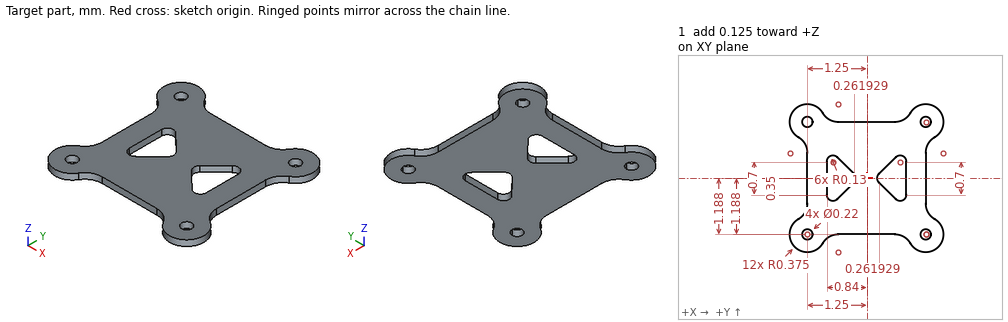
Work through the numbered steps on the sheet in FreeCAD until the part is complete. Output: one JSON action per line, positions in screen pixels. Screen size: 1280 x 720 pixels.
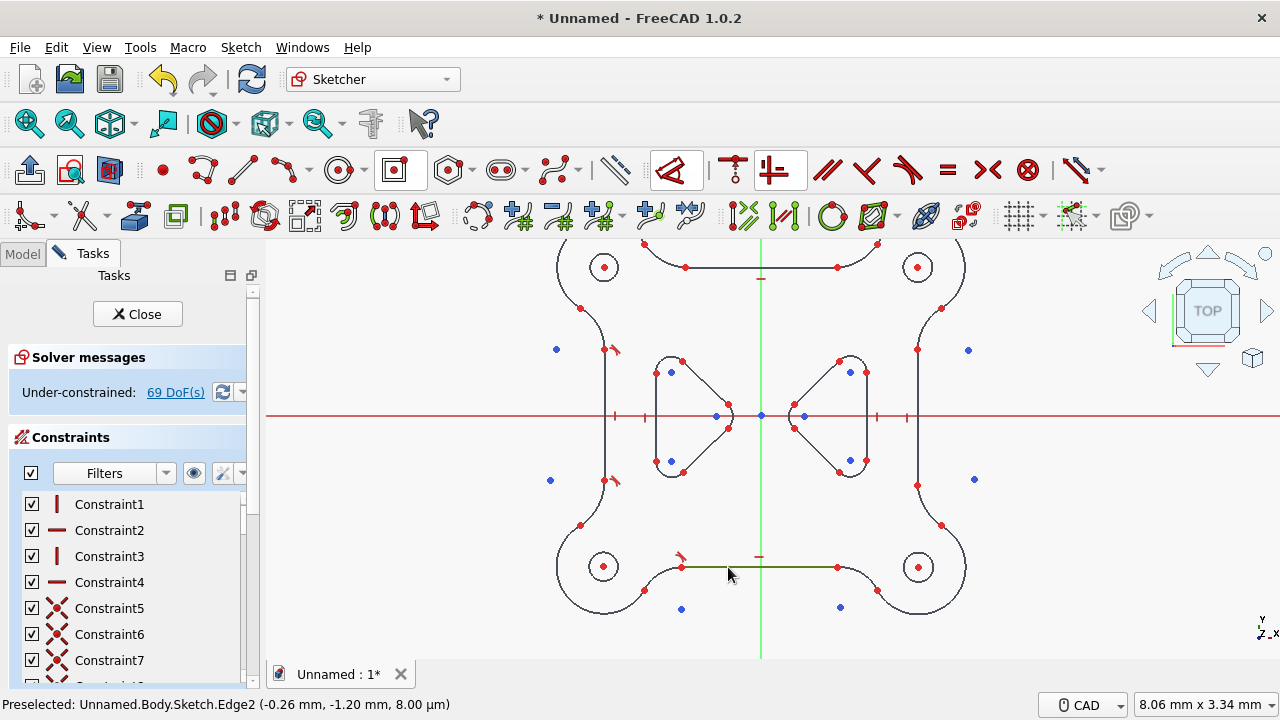
{"action": "left_click", "coordinate": [869, 578]}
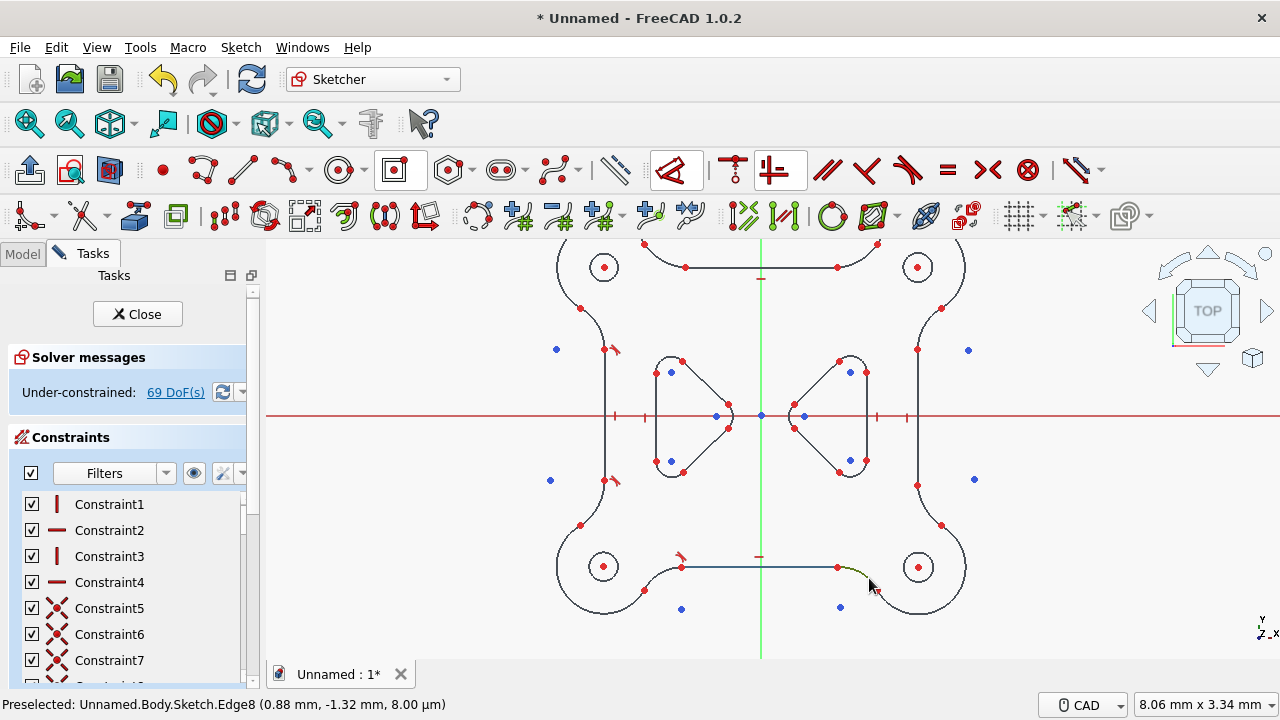
{"action": "left_click", "coordinate": [908, 170]}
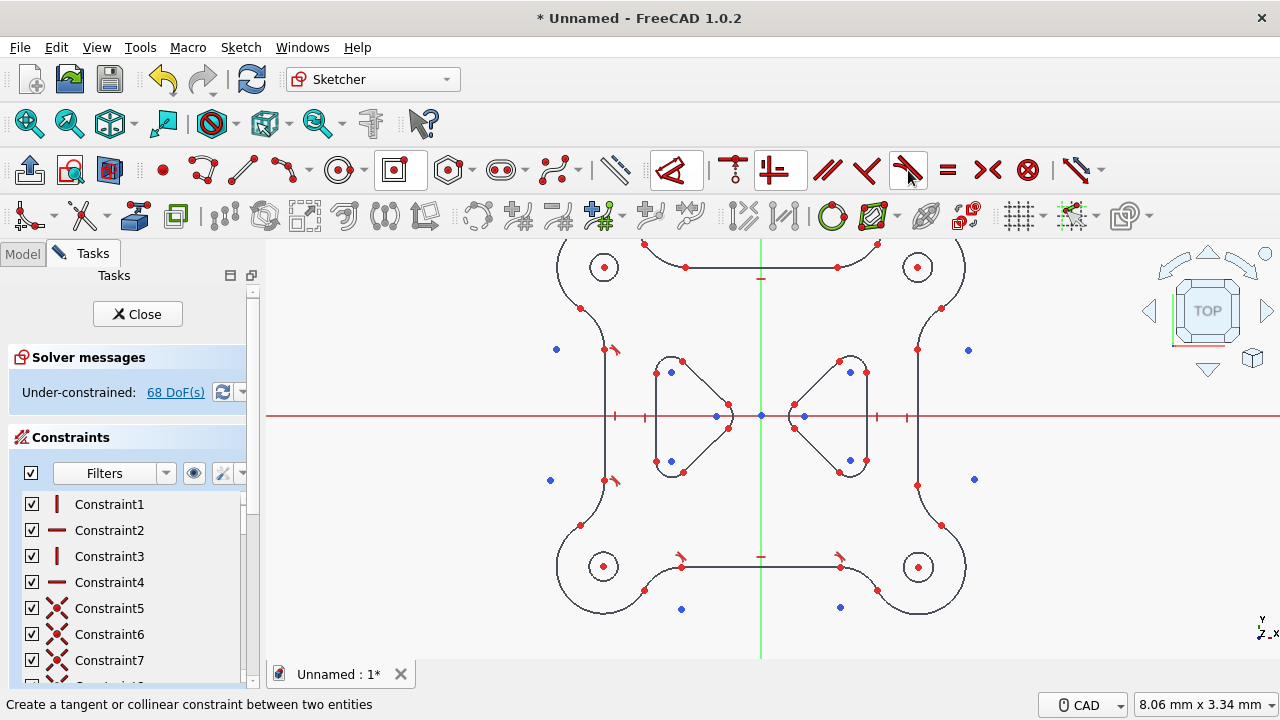
{"action": "left_click", "coordinate": [918, 445]}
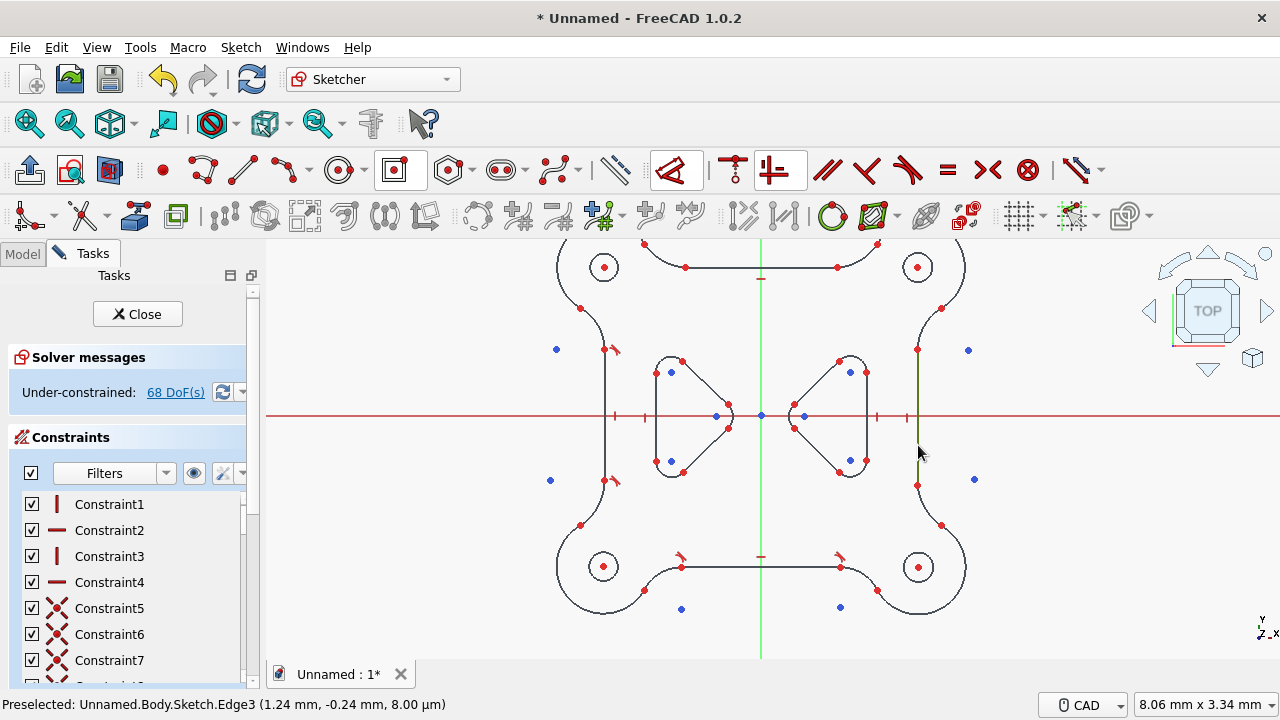
{"action": "left_click", "coordinate": [921, 500]}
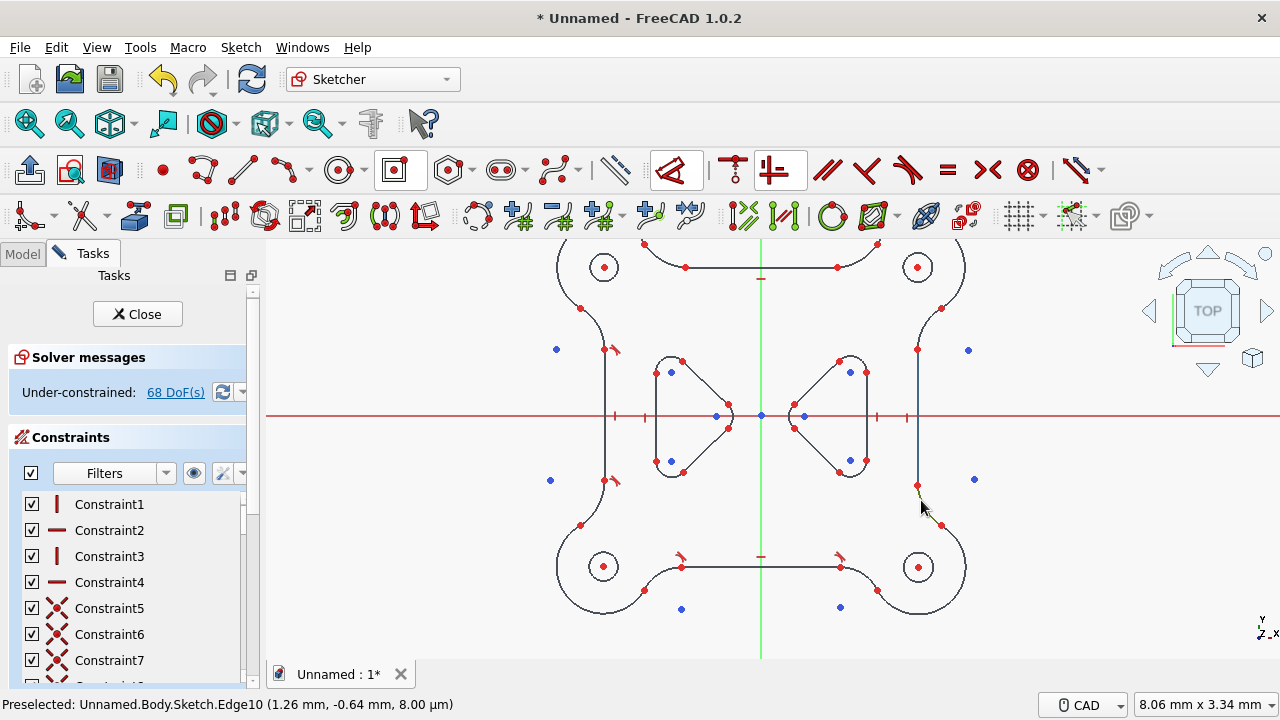
{"action": "left_click", "coordinate": [908, 170]}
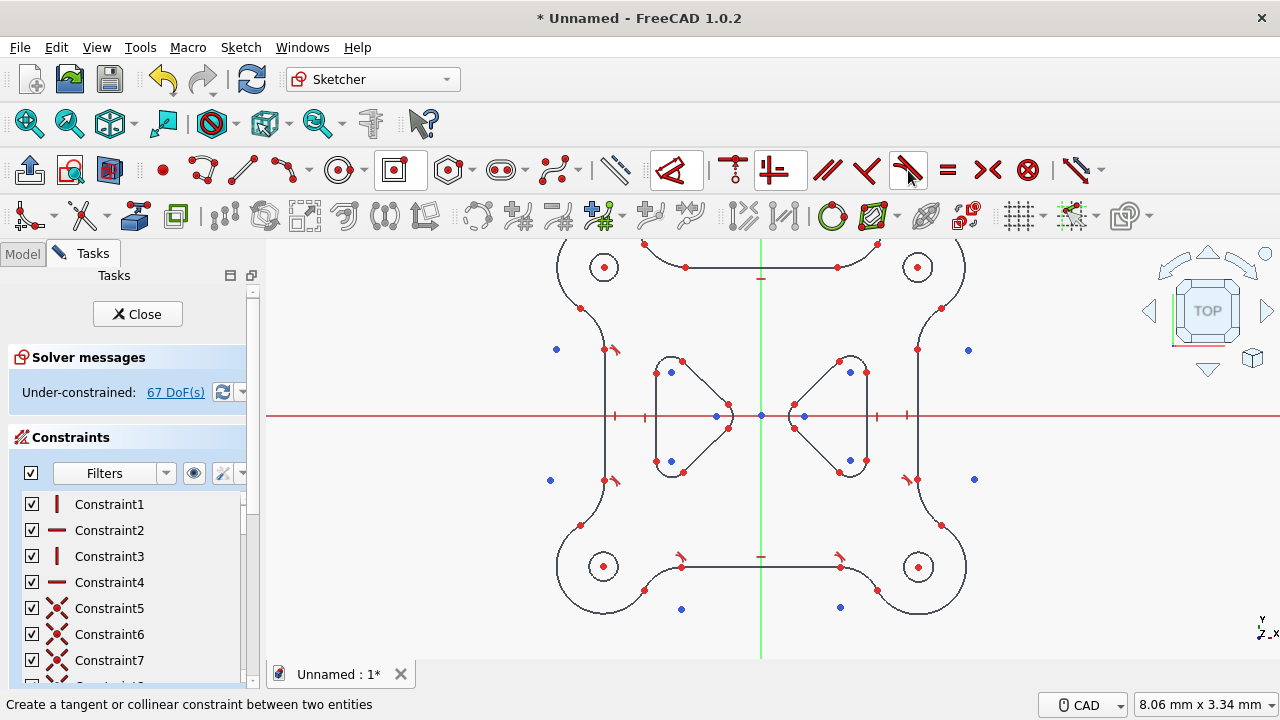
{"action": "left_click", "coordinate": [918, 440]}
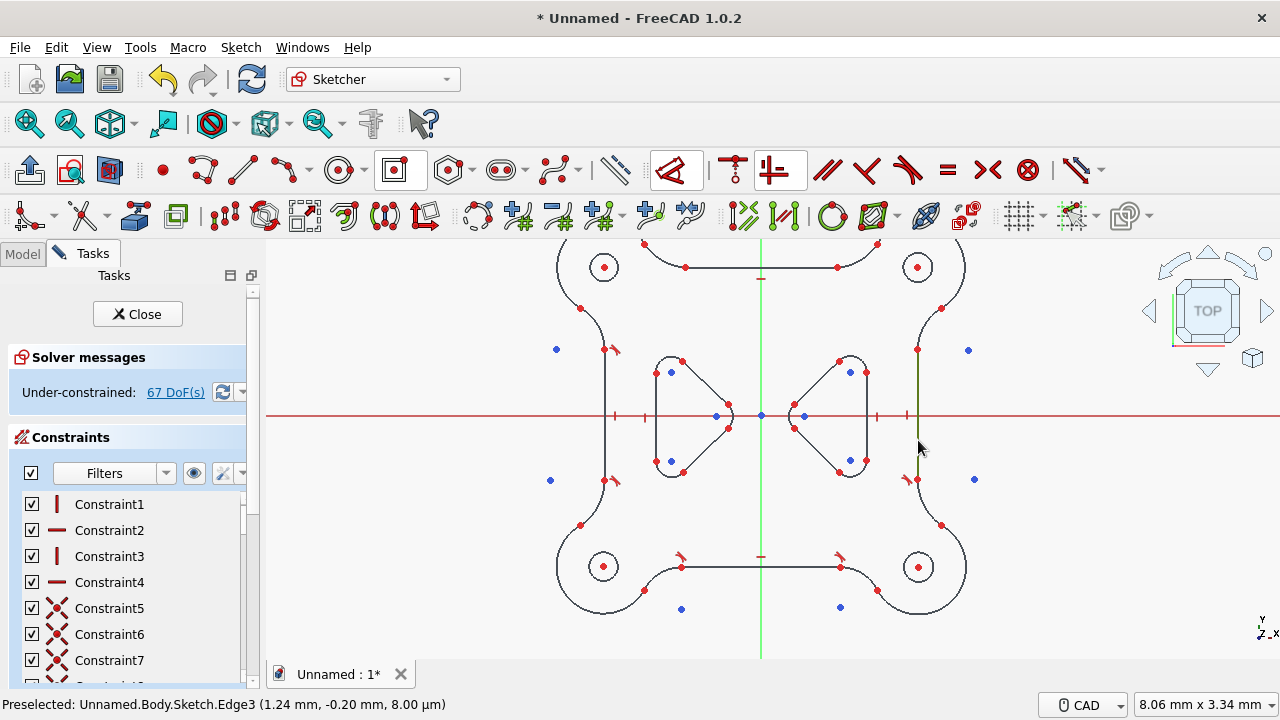
{"action": "left_click", "coordinate": [930, 318]}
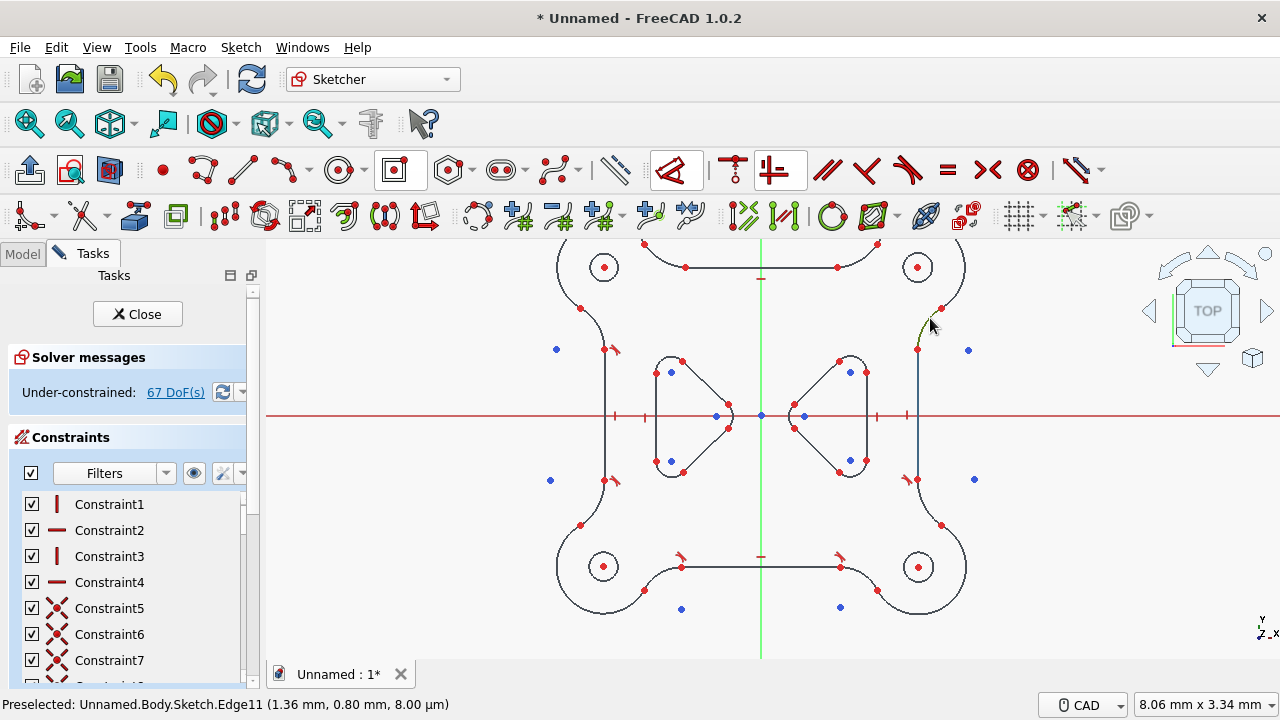
{"action": "left_click", "coordinate": [908, 170]}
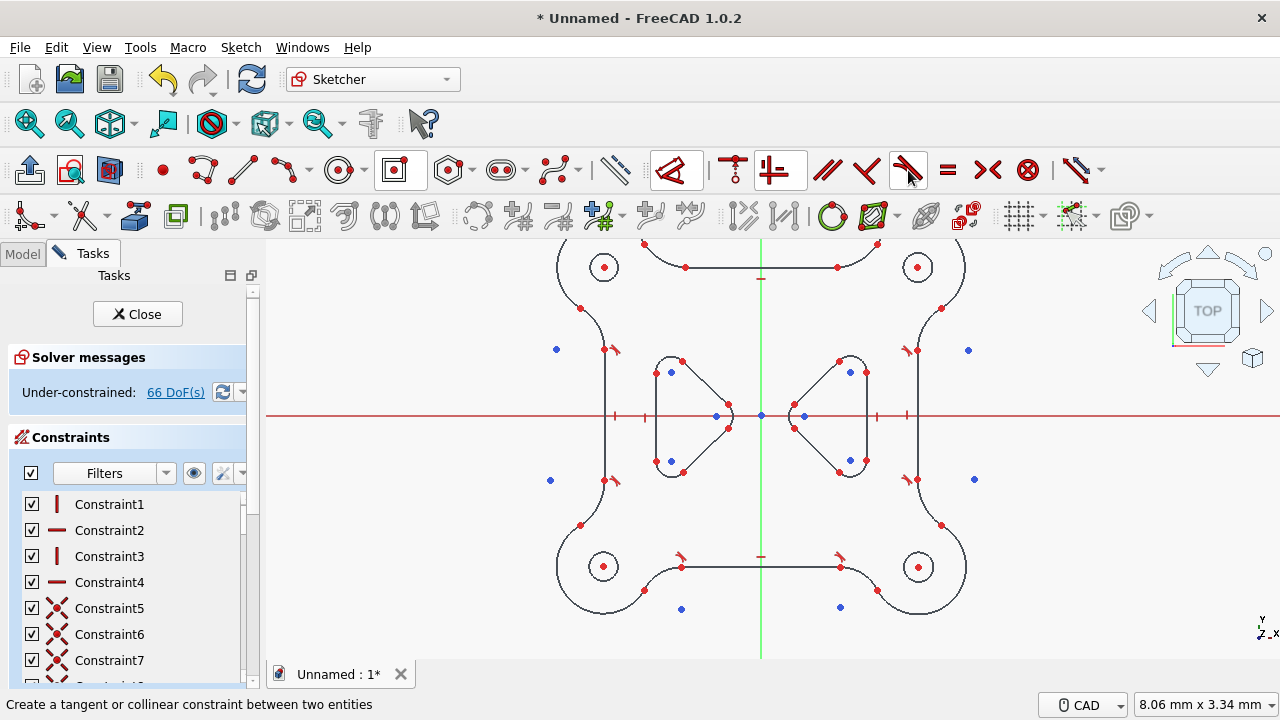
{"action": "left_click", "coordinate": [792, 268]}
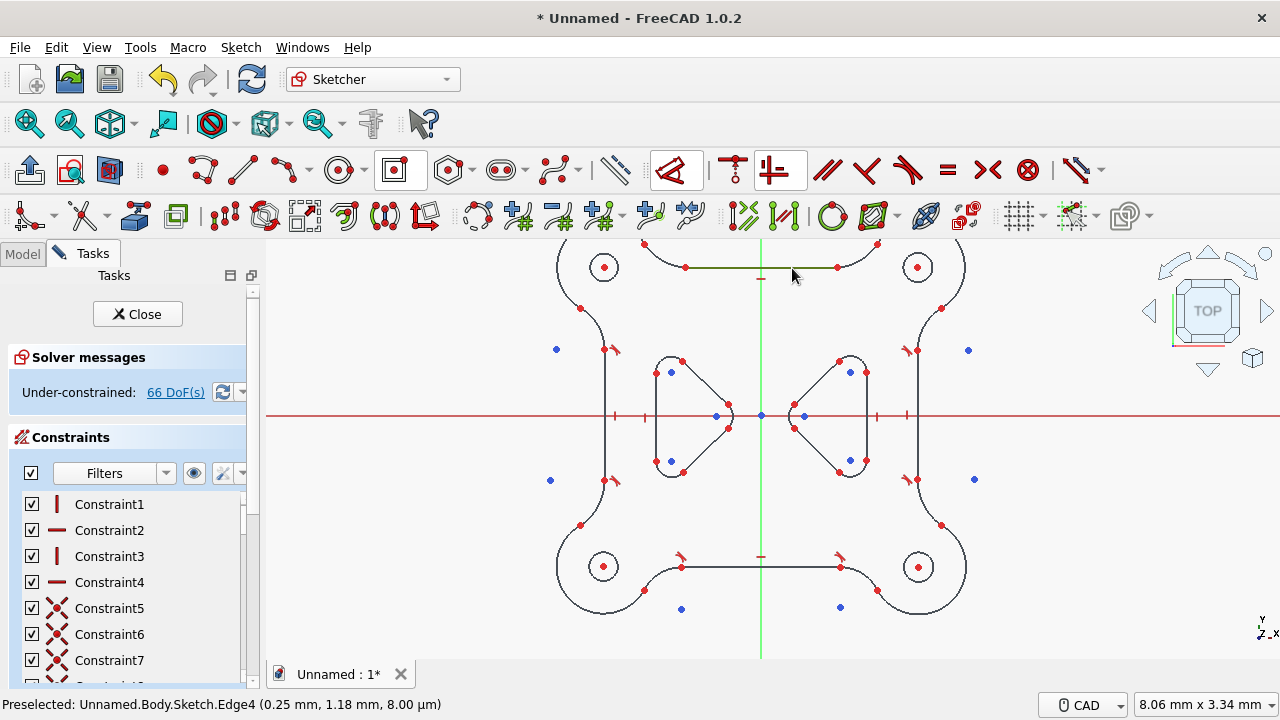
{"action": "scroll", "coordinate": [590, 516], "scroll_direction": "down", "scroll_amount": 2}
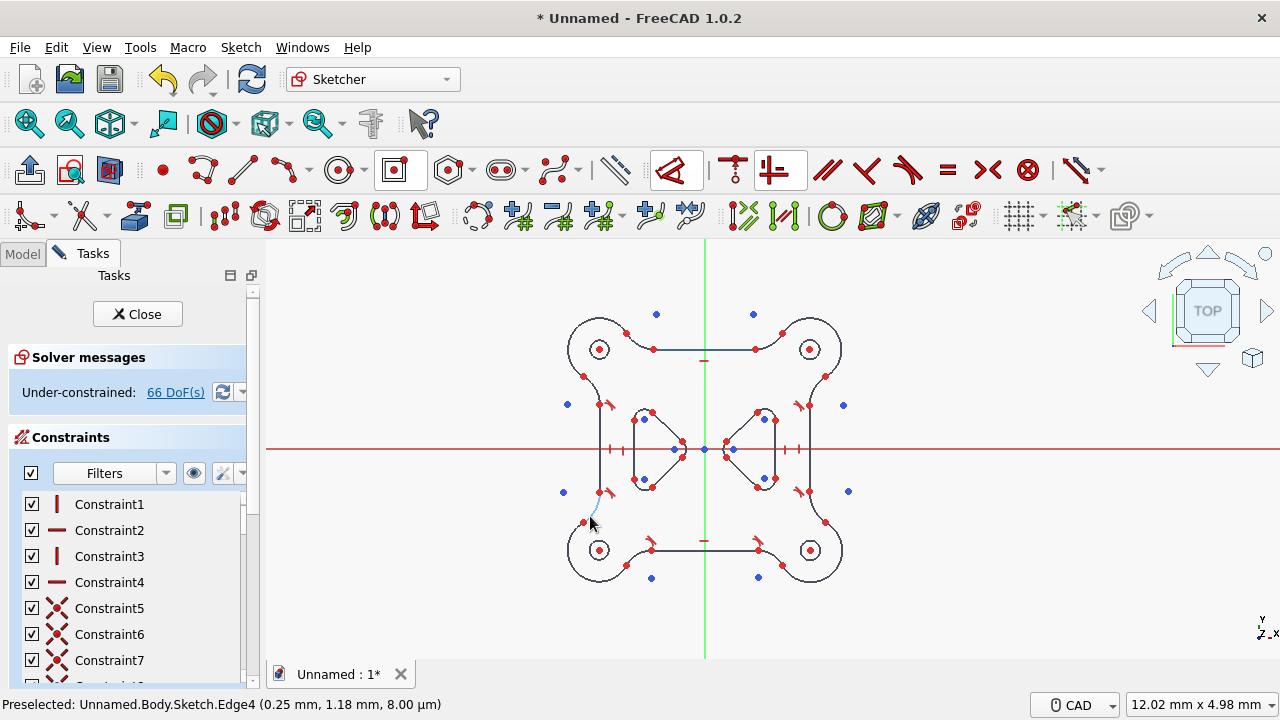
{"action": "scroll", "coordinate": [765, 348], "scroll_direction": "up", "scroll_amount": 2}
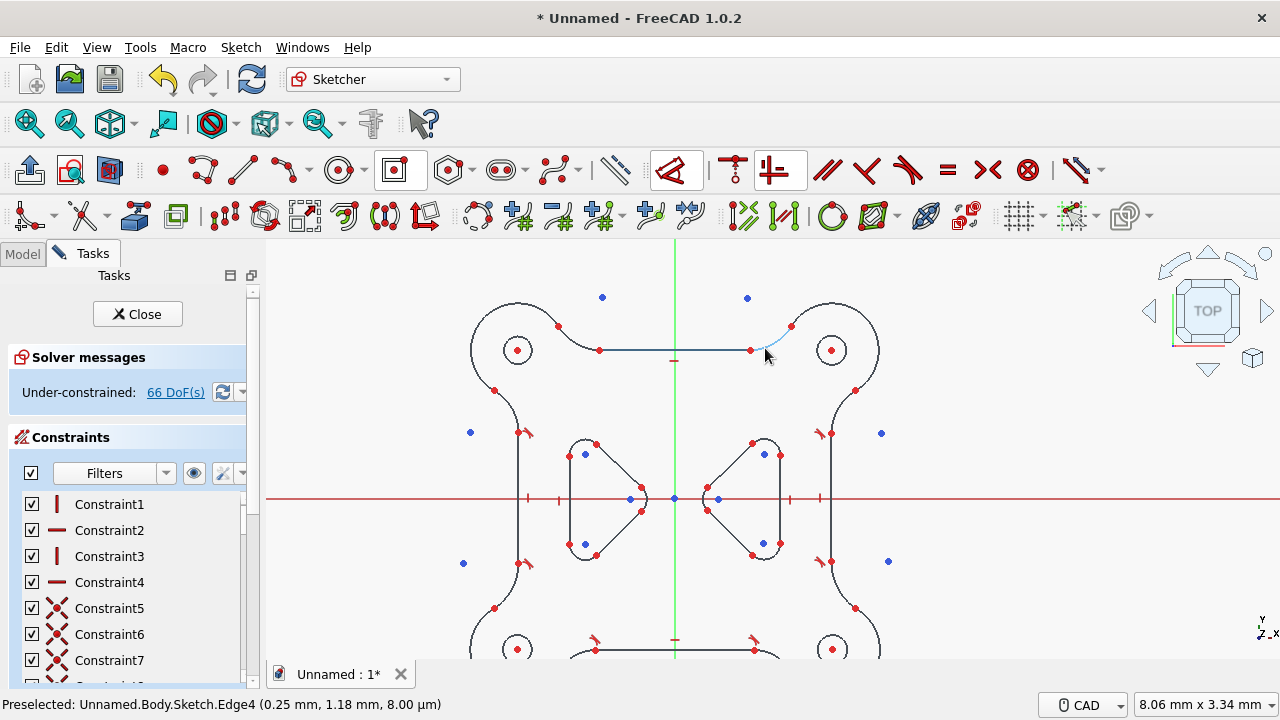
{"action": "left_click", "coordinate": [765, 347]}